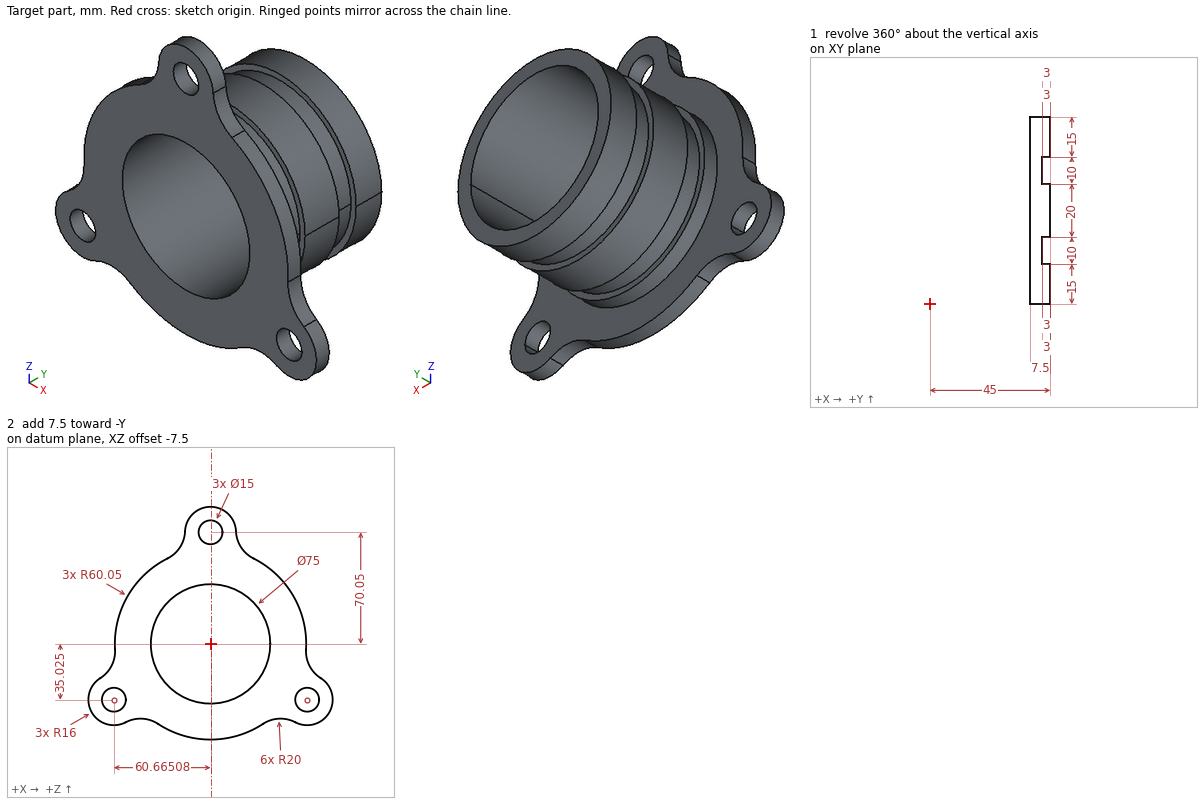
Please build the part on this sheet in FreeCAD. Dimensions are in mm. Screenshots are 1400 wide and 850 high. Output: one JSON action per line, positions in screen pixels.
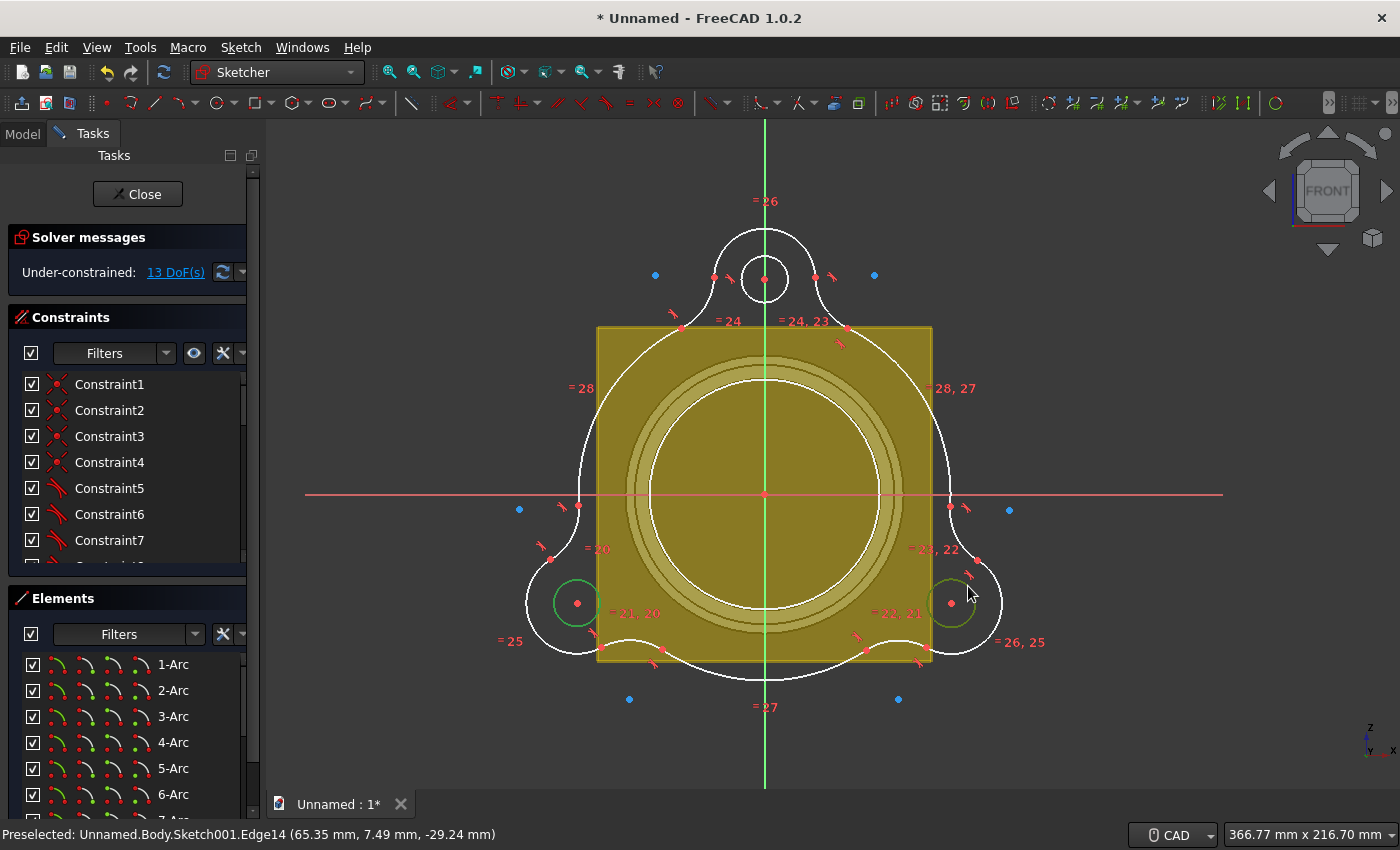
{"action": "left_click", "coordinate": [781, 263]}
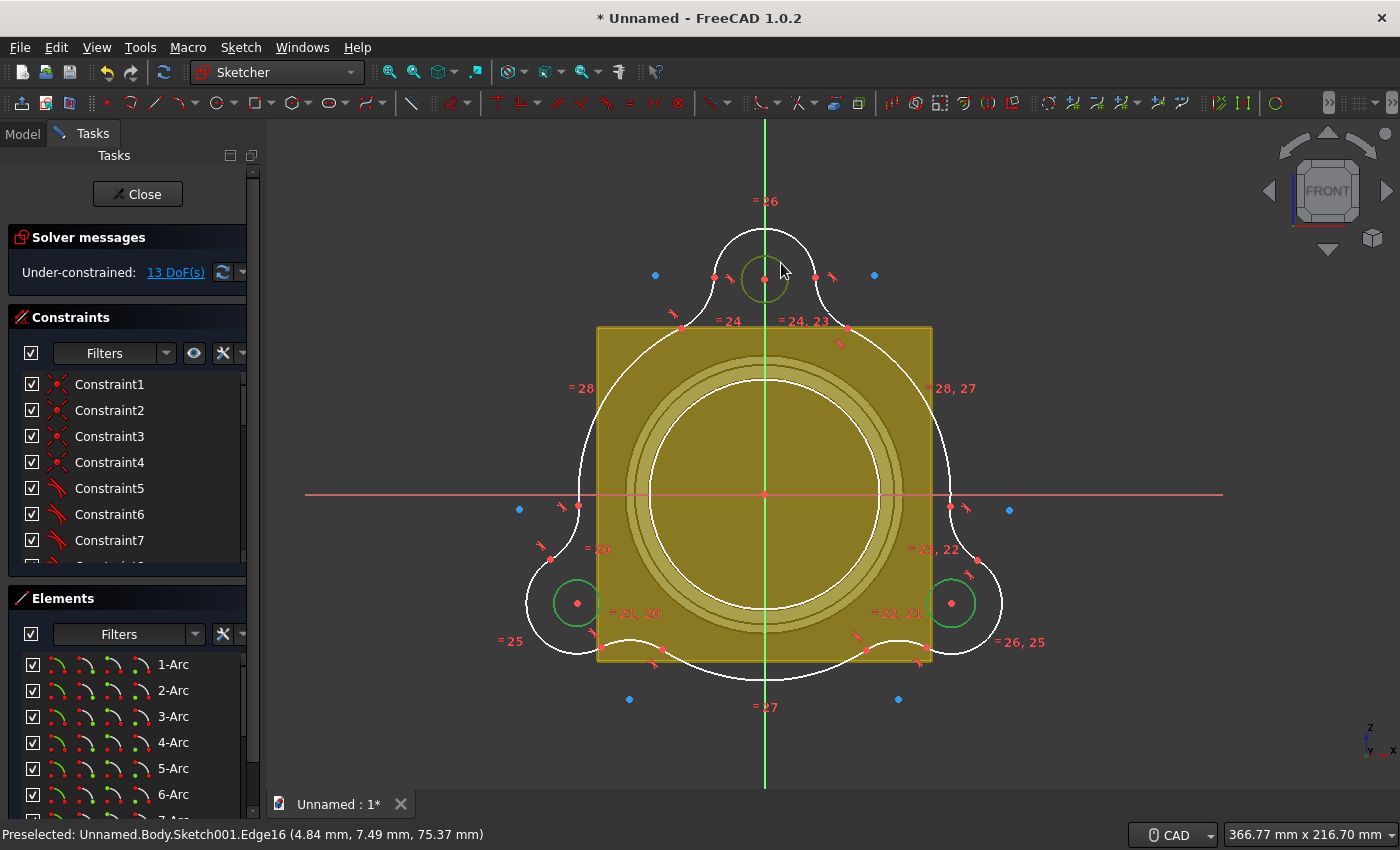
{"action": "left_click", "coordinate": [630, 104]}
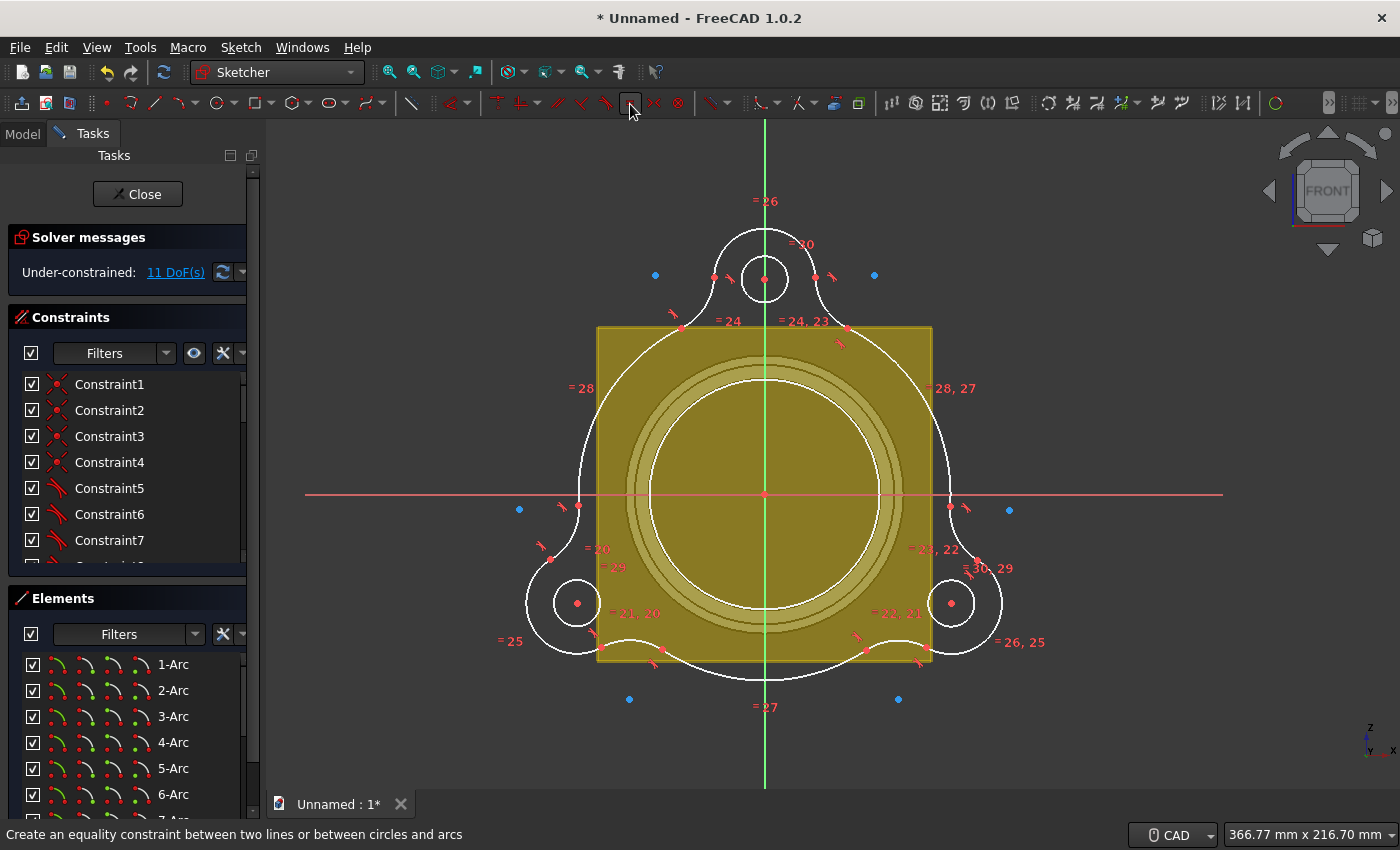
{"action": "left_click", "coordinate": [765, 279]}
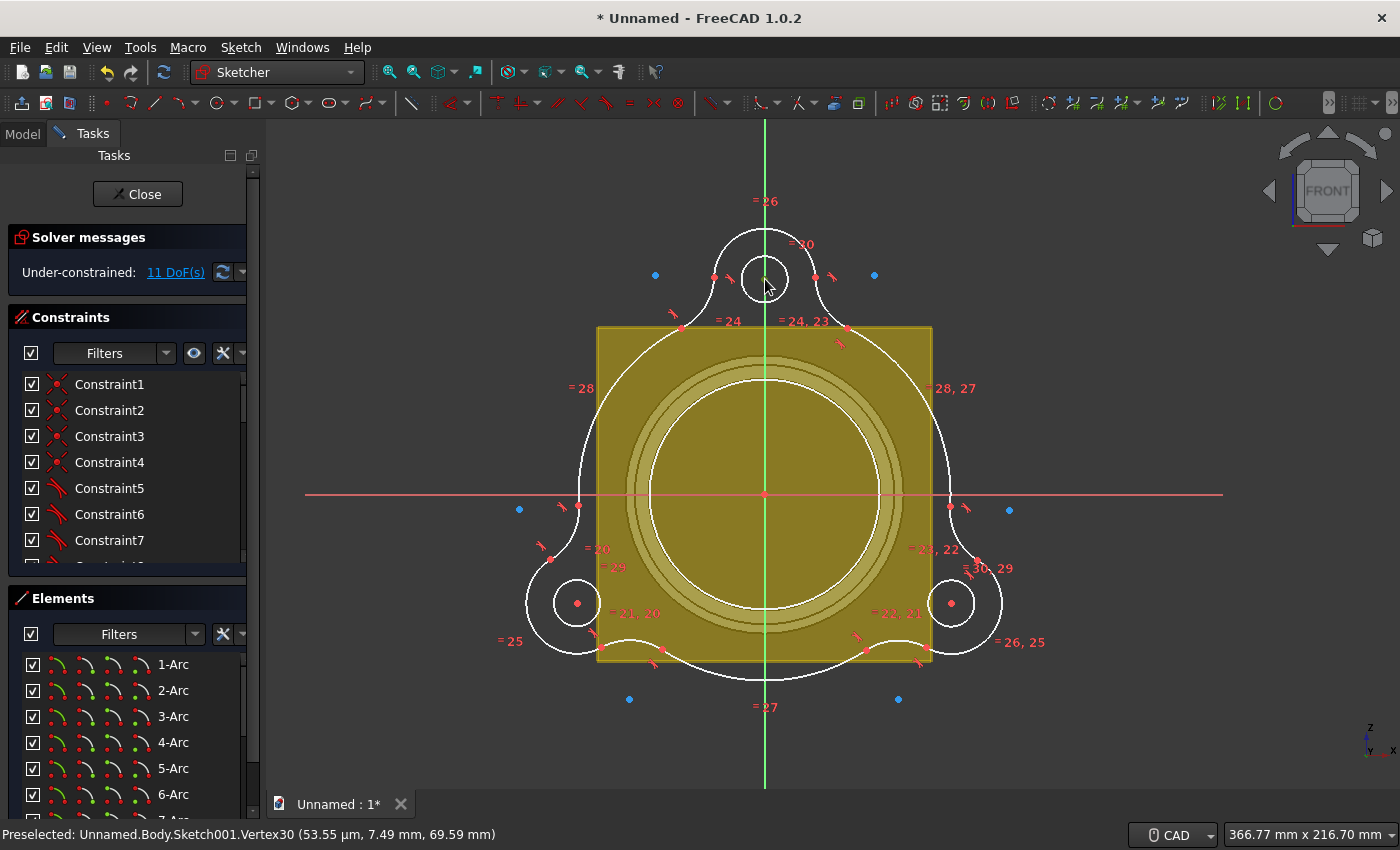
{"action": "left_click", "coordinate": [765, 717]}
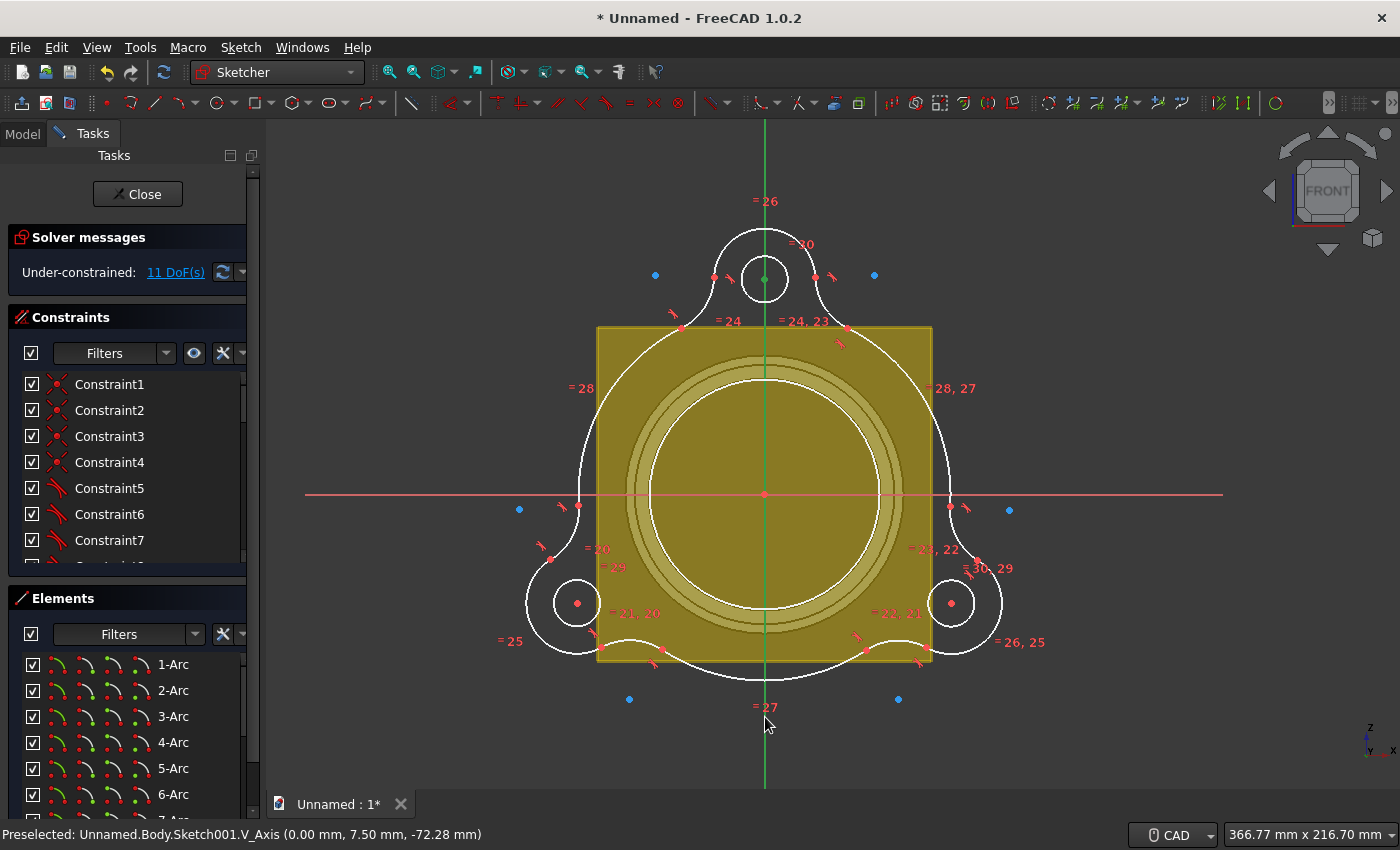
{"action": "left_click", "coordinate": [498, 104]}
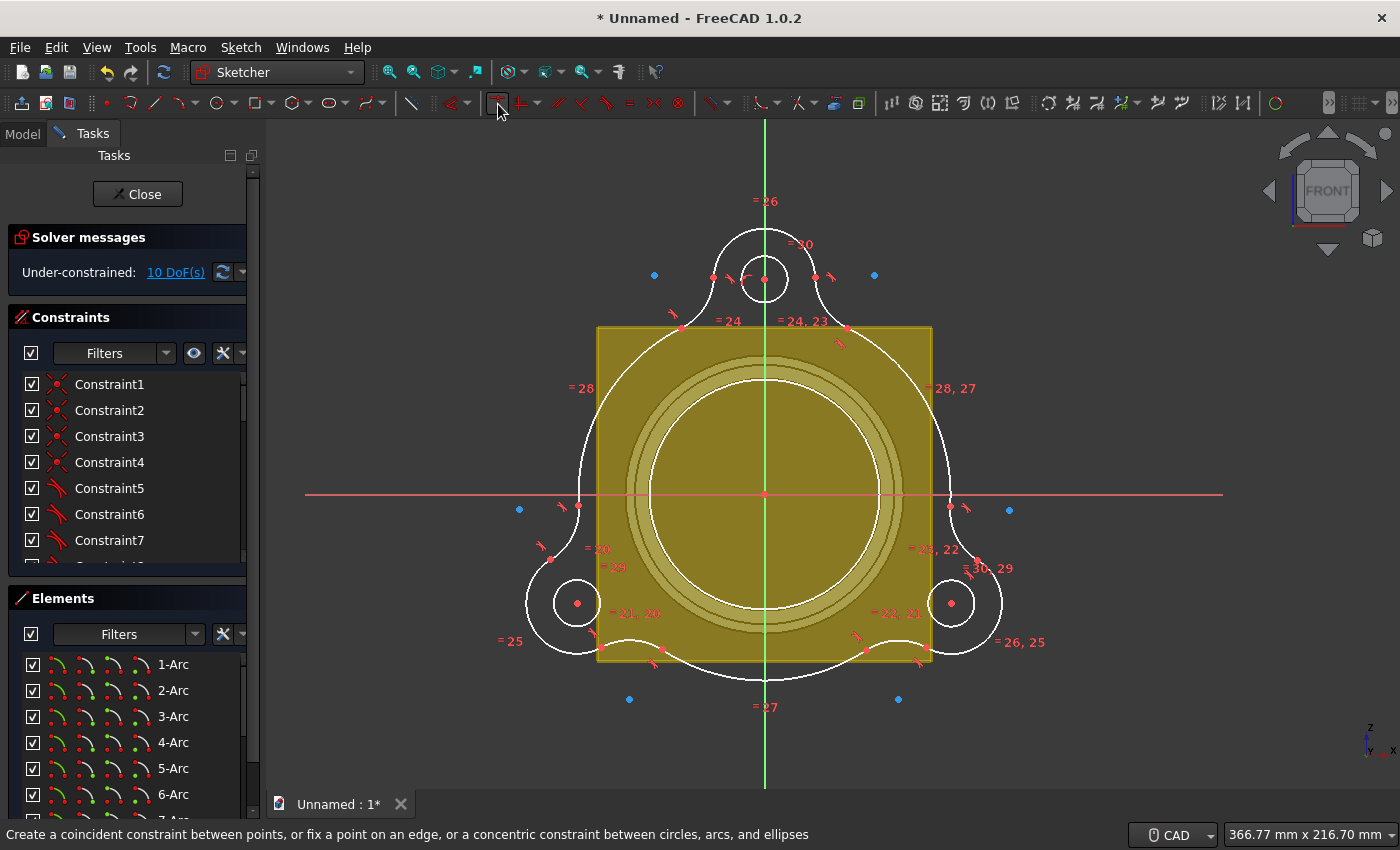
{"action": "left_click", "coordinate": [577, 603]}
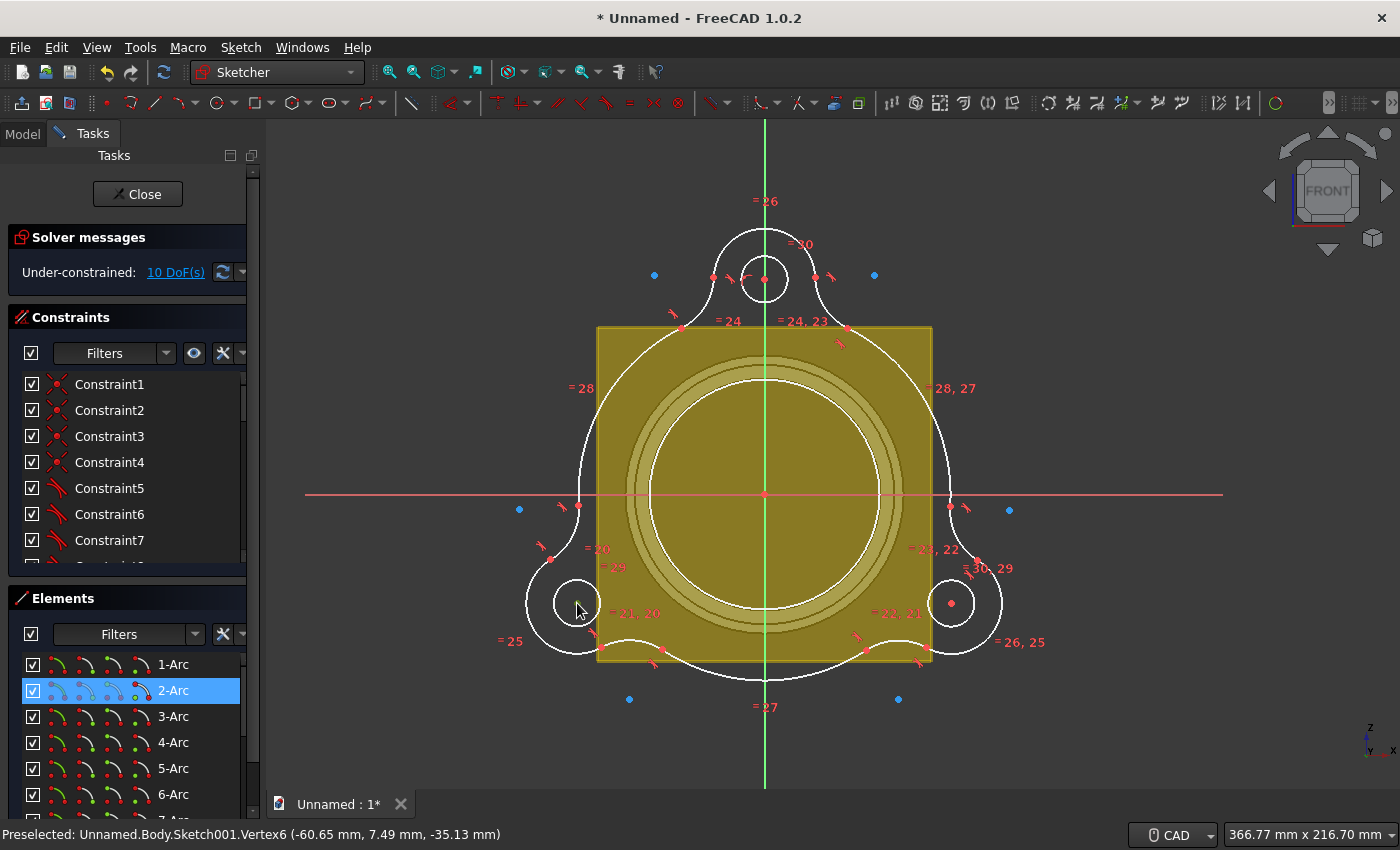
{"action": "left_click", "coordinate": [951, 603]}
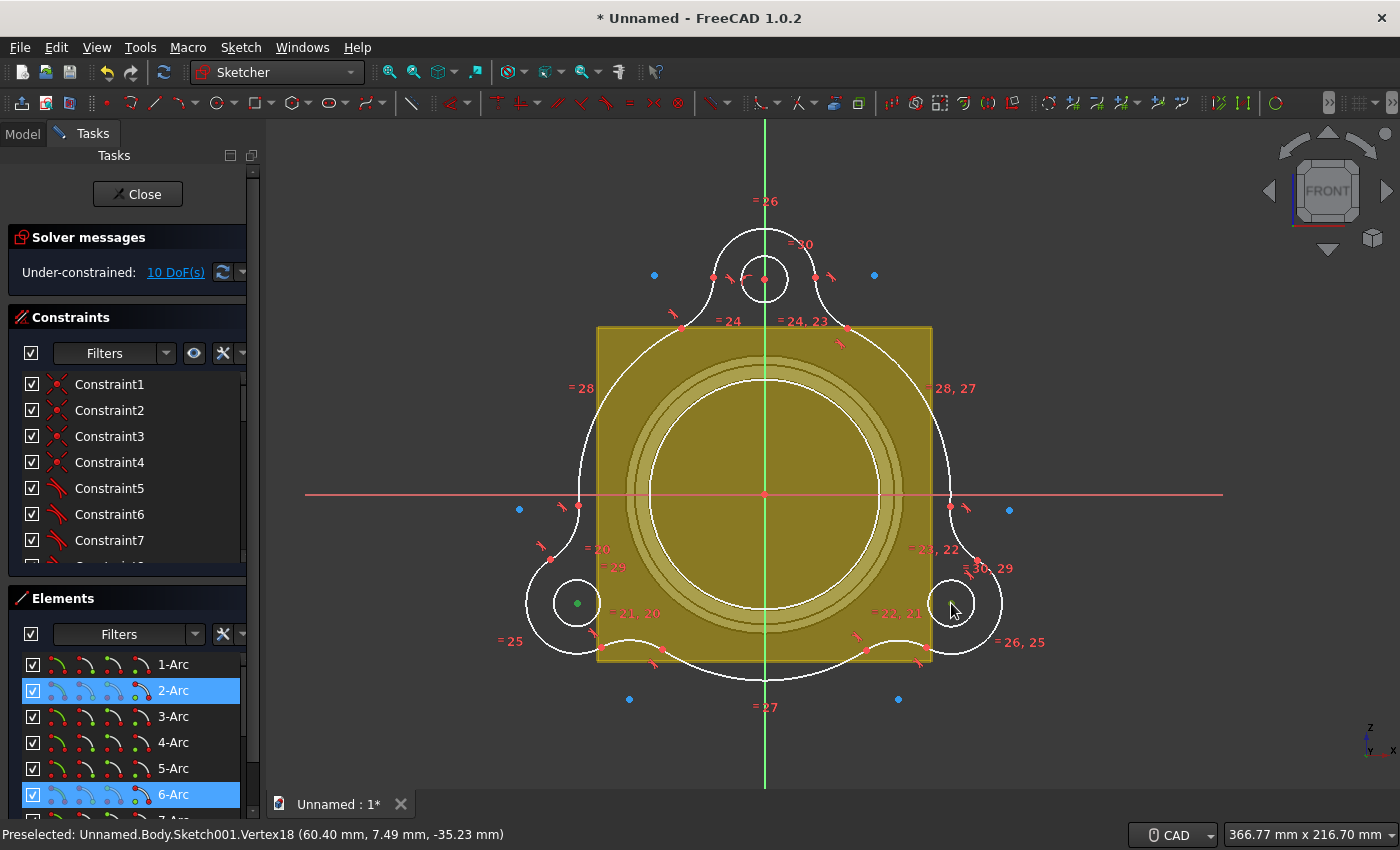
{"action": "left_click", "coordinate": [765, 717]}